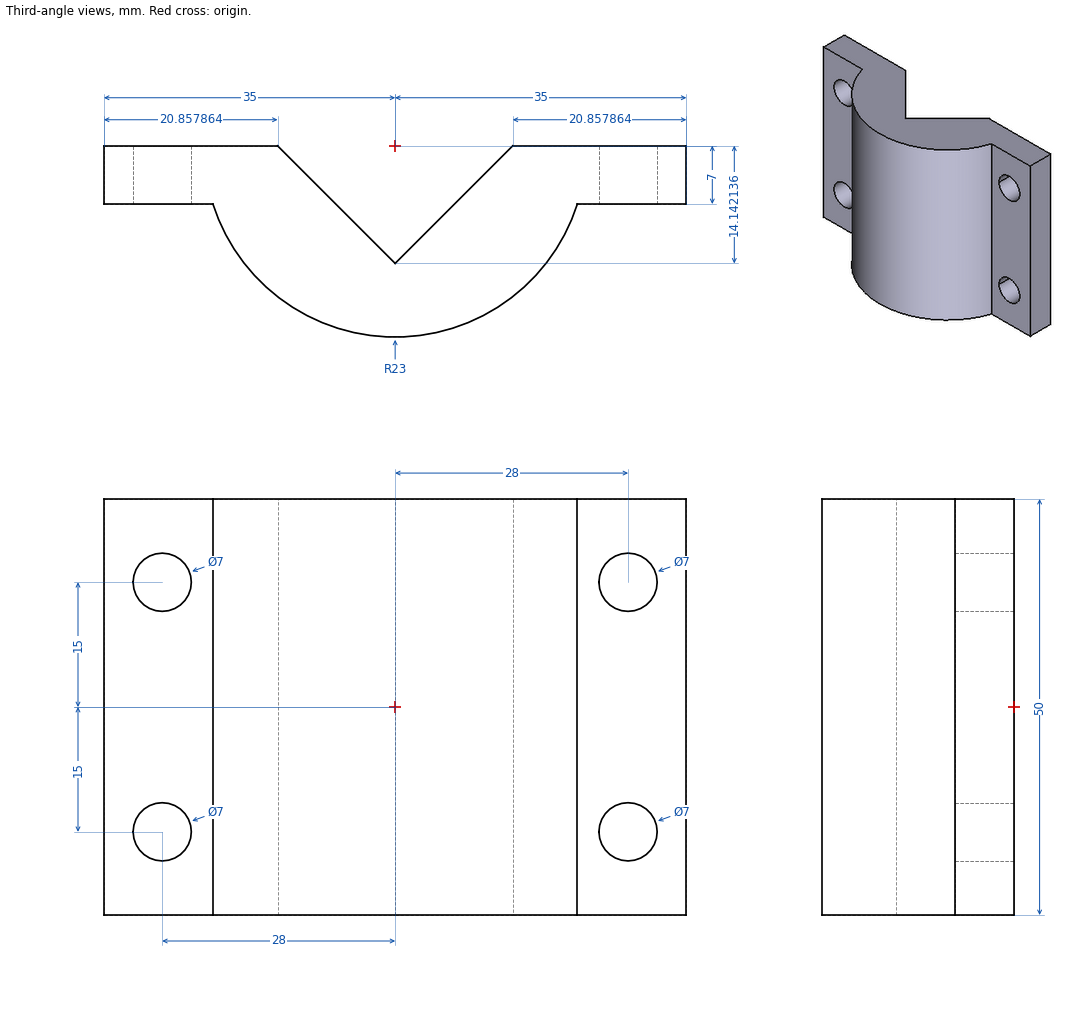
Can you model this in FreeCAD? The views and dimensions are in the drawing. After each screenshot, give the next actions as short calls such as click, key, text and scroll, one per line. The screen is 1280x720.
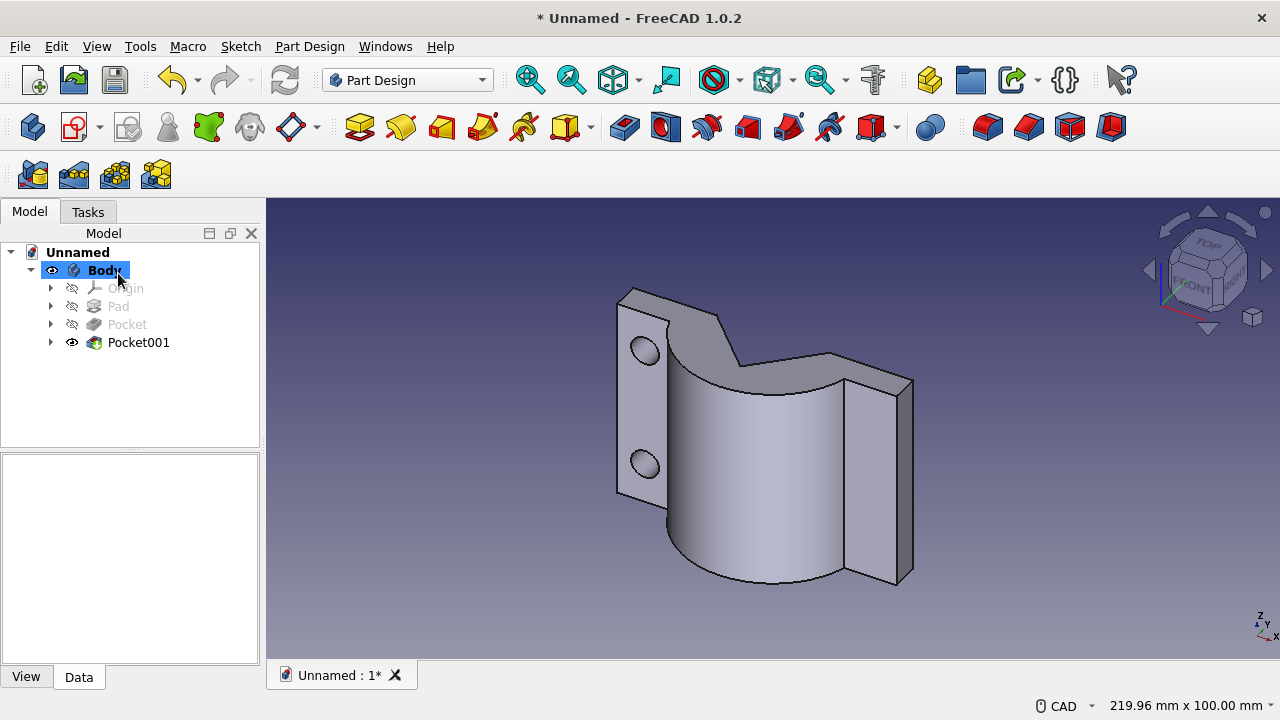
key(4)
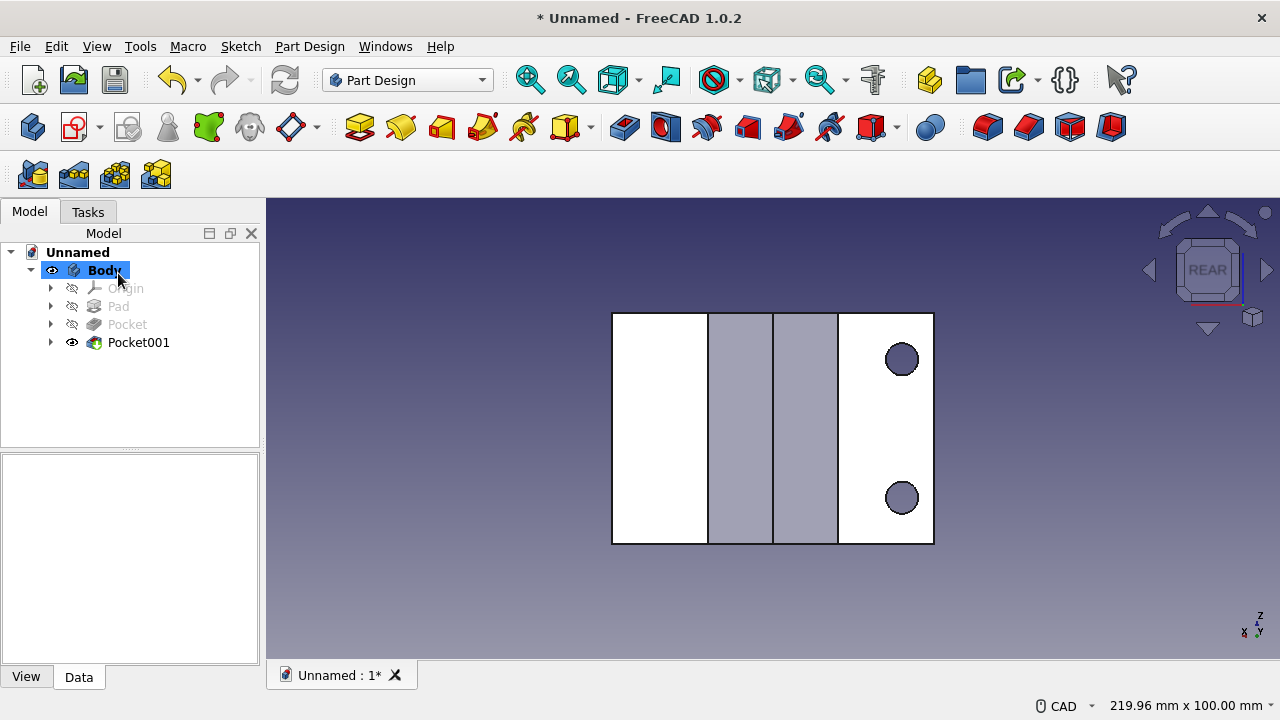
click(660, 362)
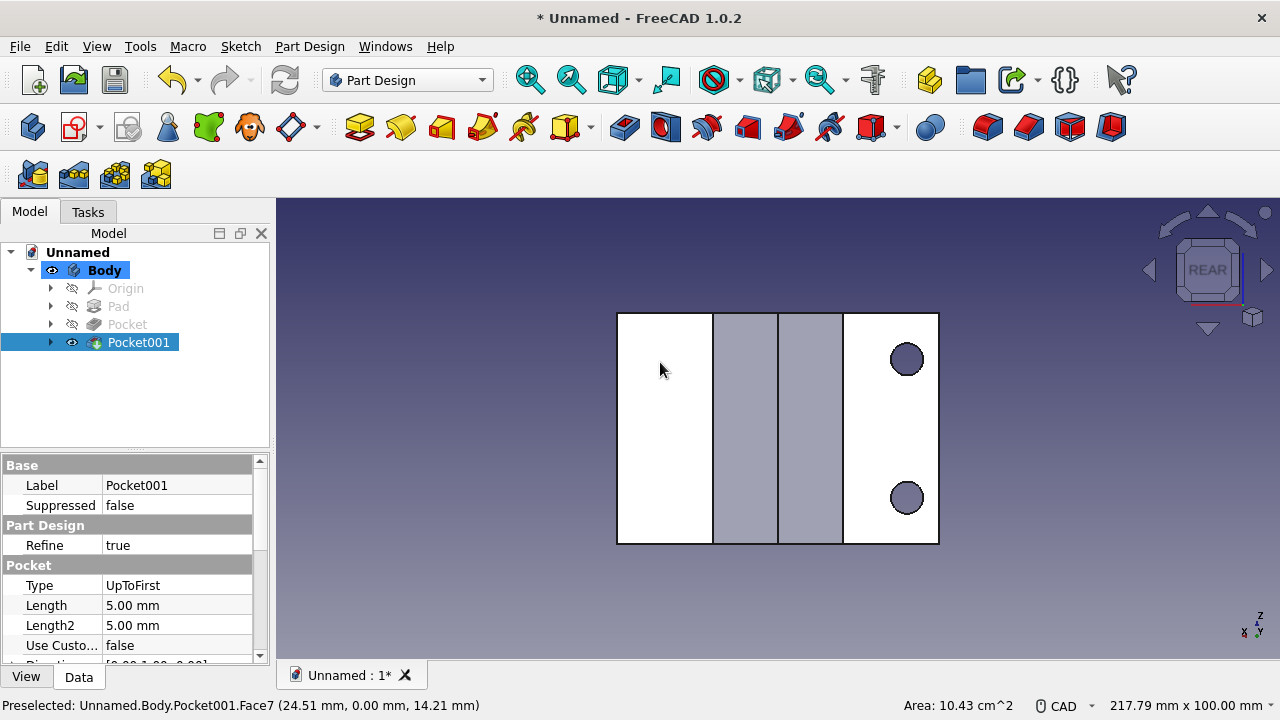
click(74, 128)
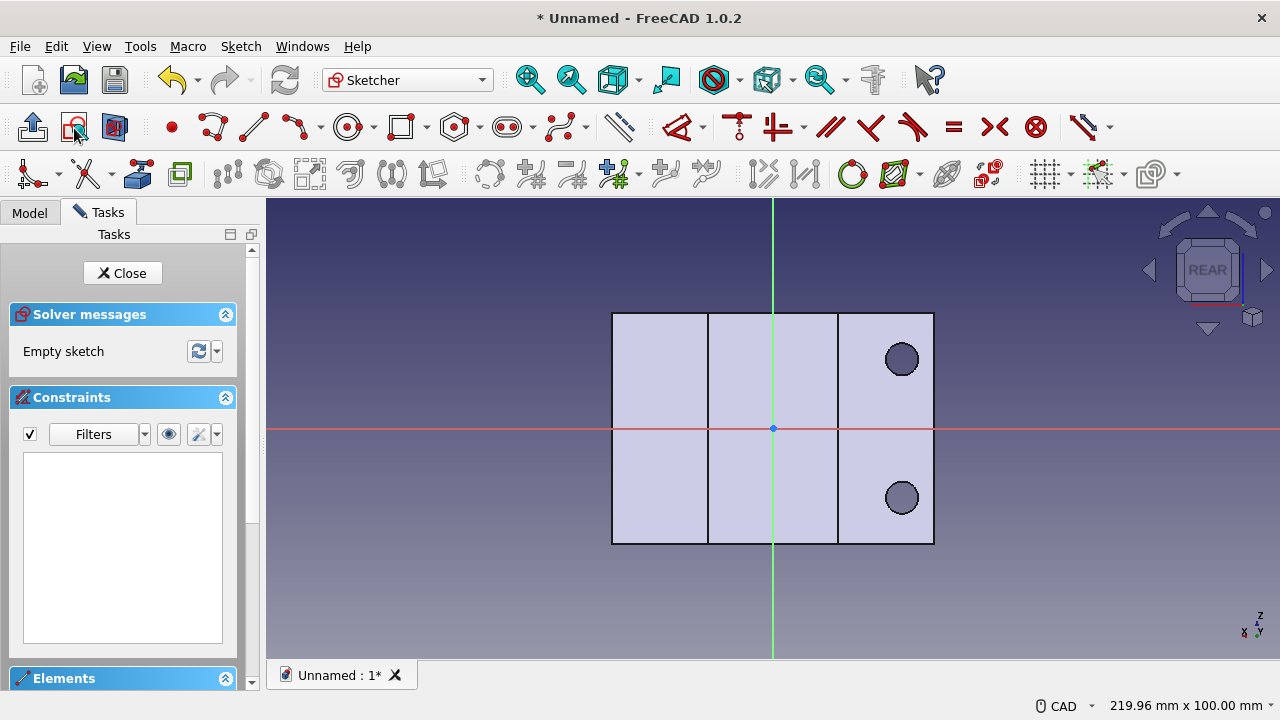
scroll(636, 351, up, 11)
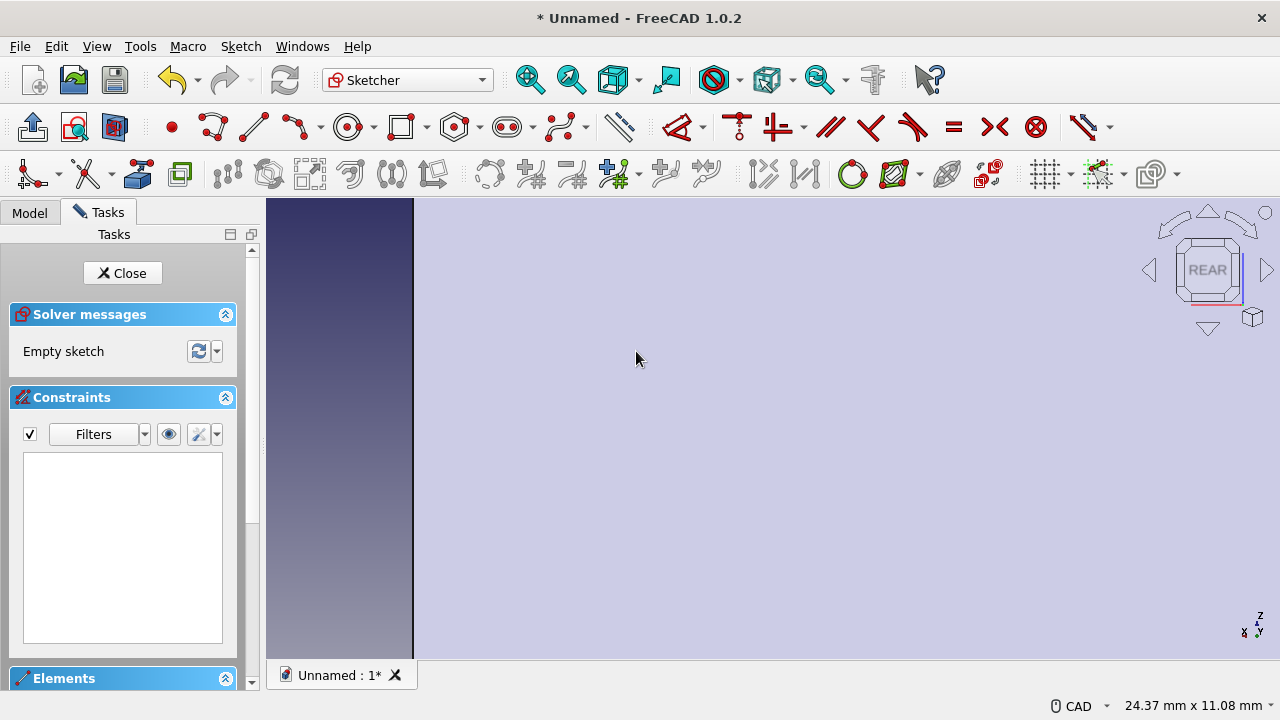
click(348, 128)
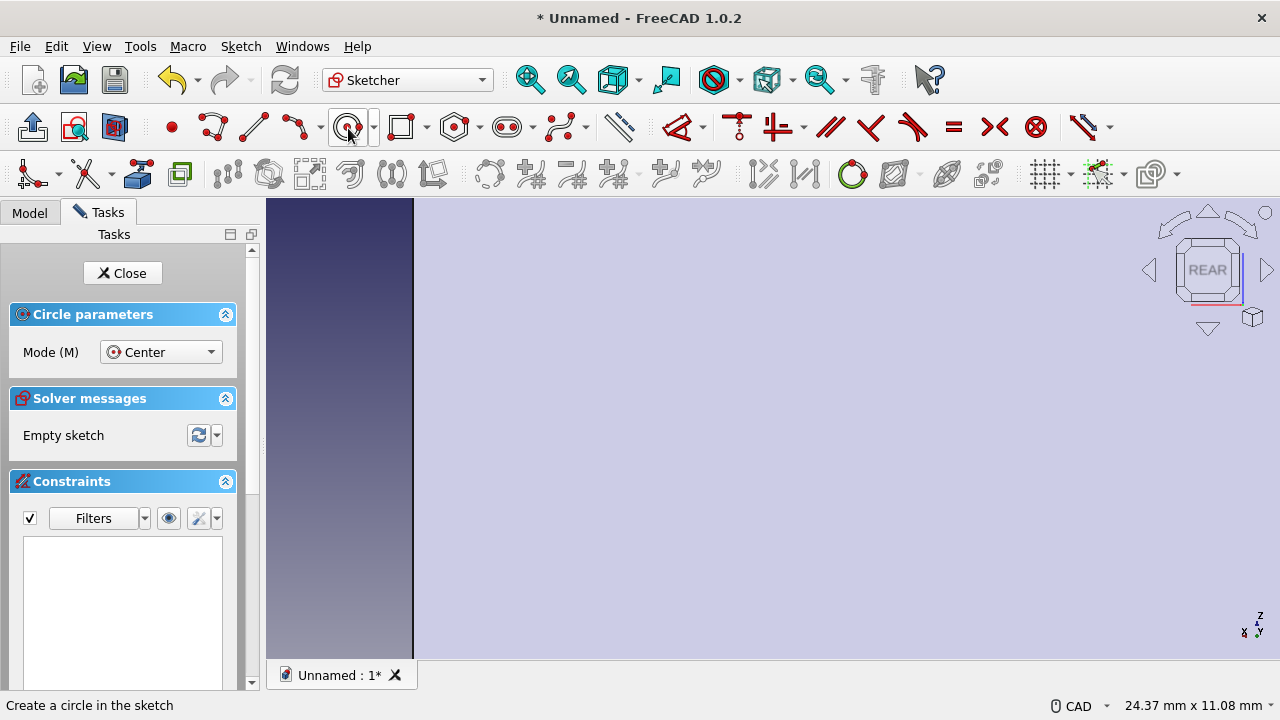
click(705, 424)
click(808, 321)
key(Escape)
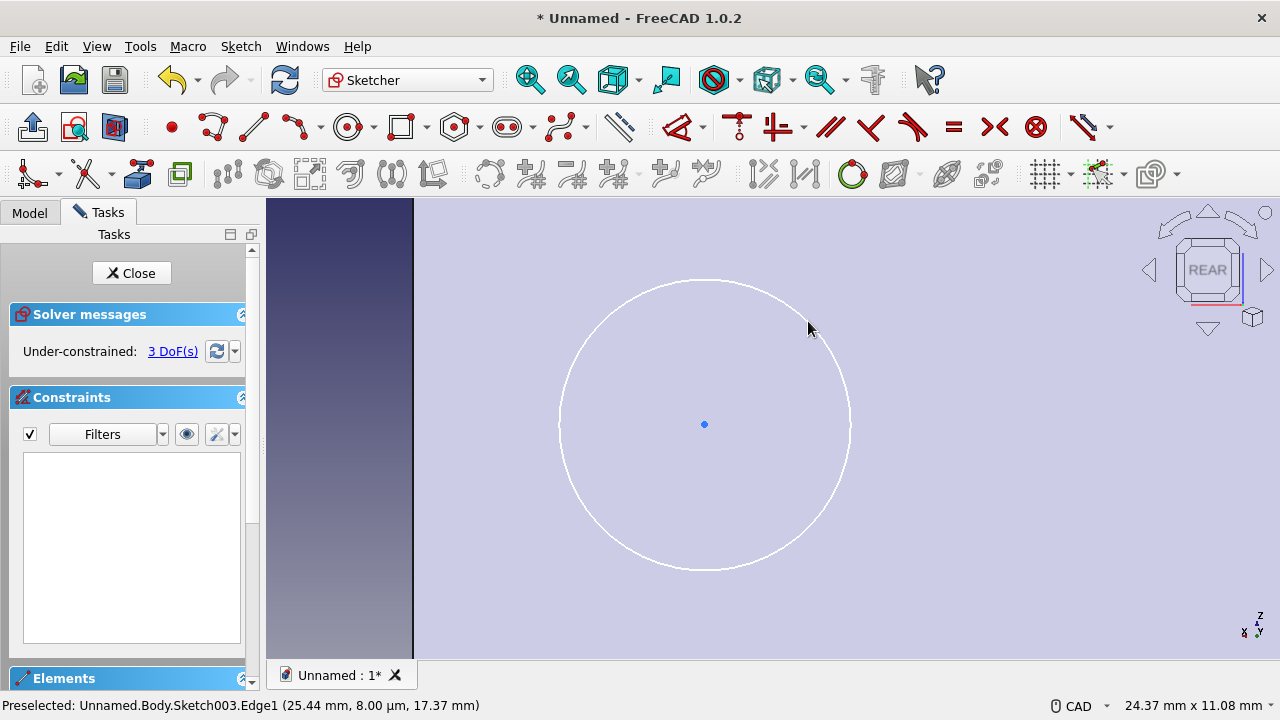
key(d)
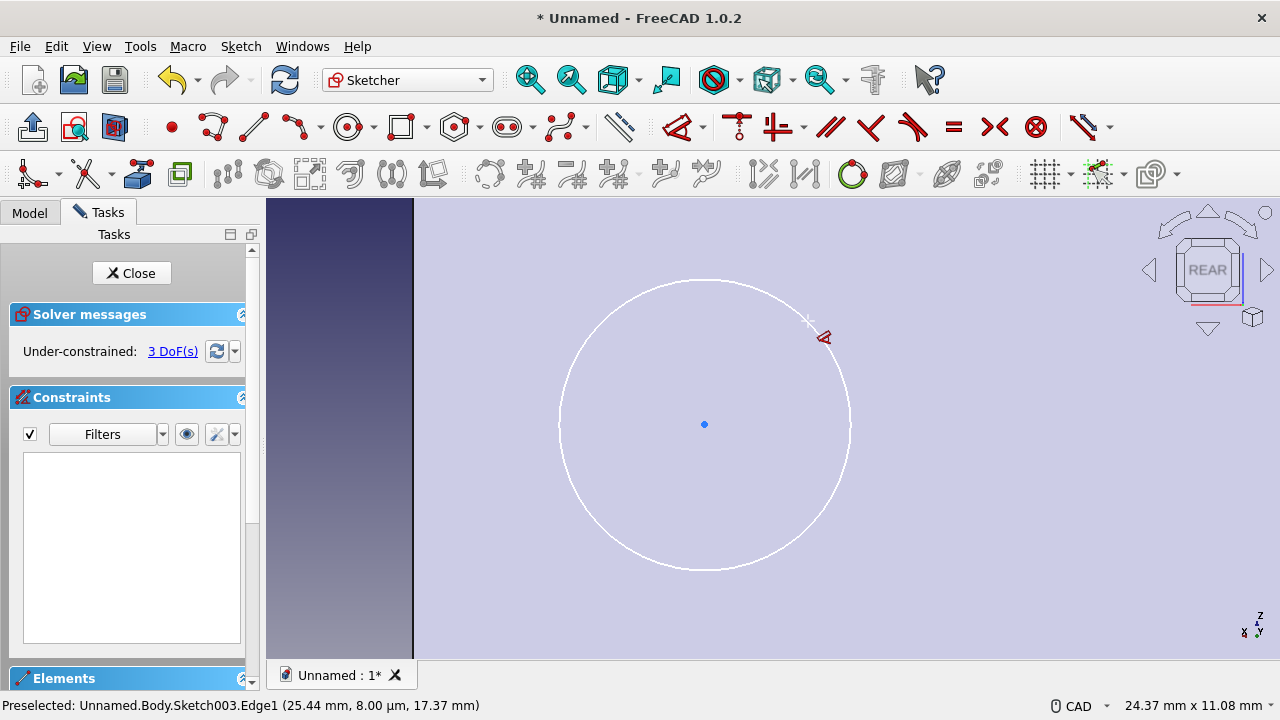
click(808, 322)
click(831, 299)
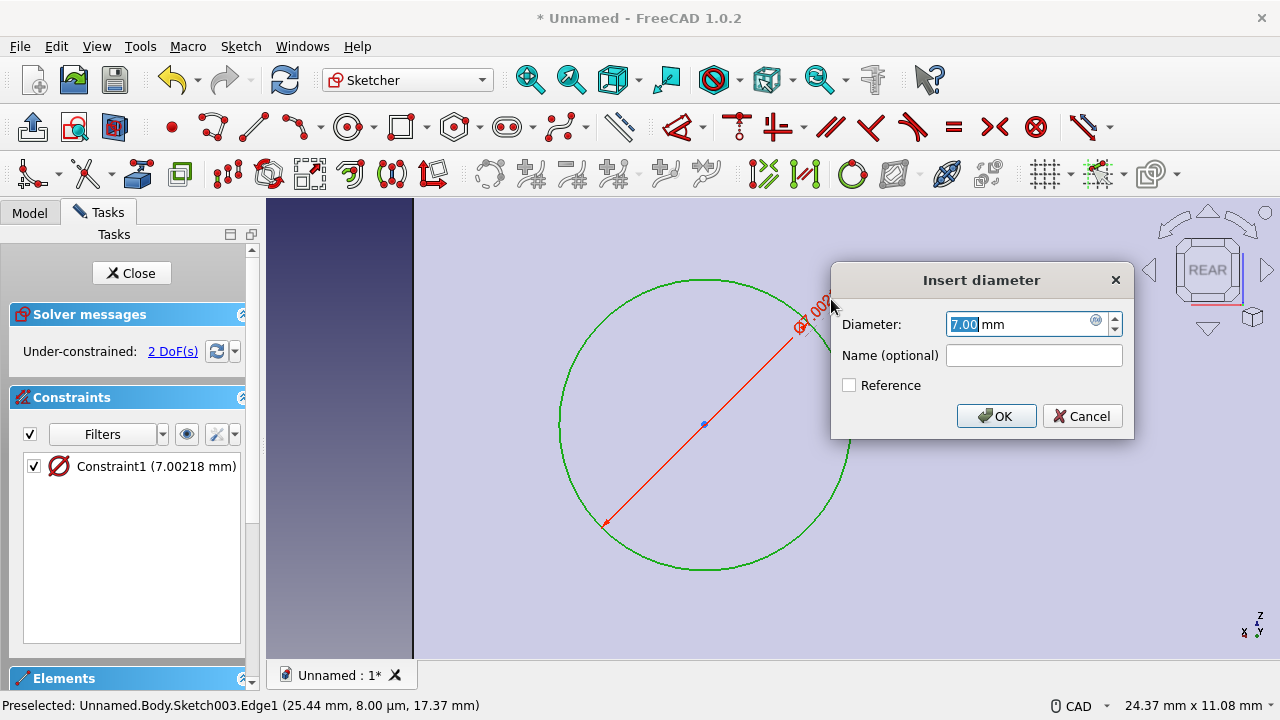
text(7)
key(Return)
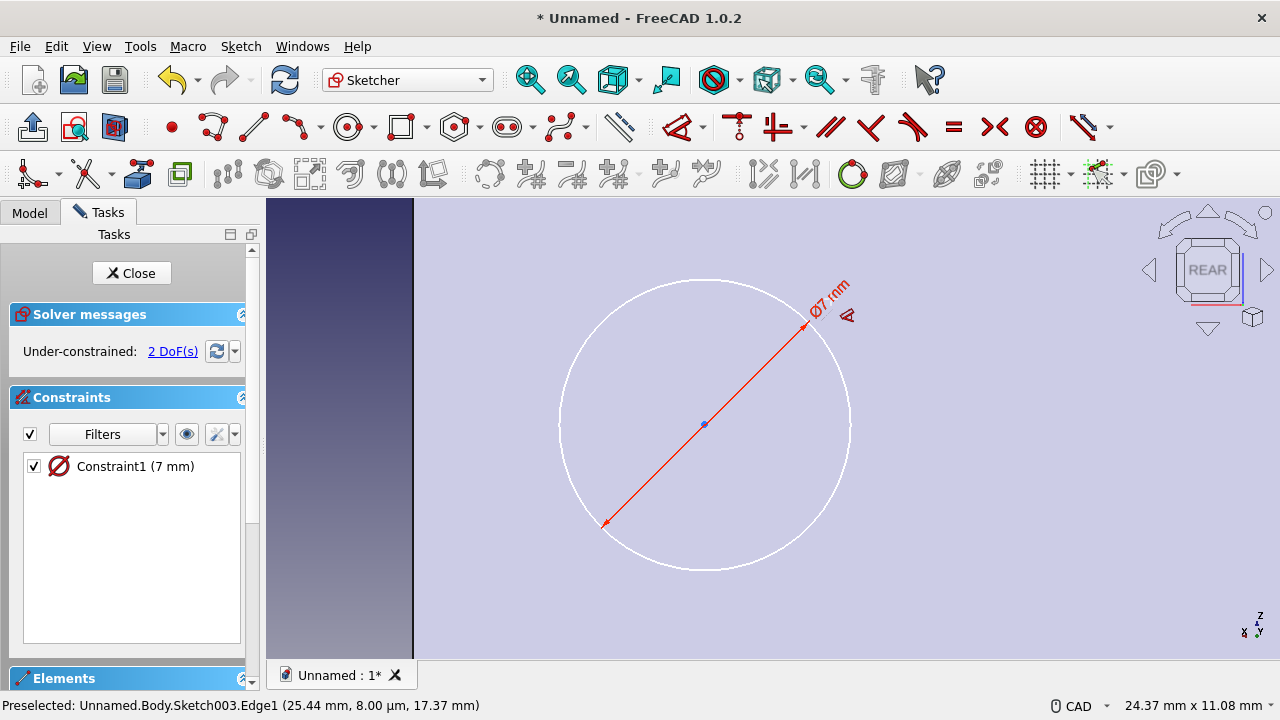
click(705, 425)
click(910, 391)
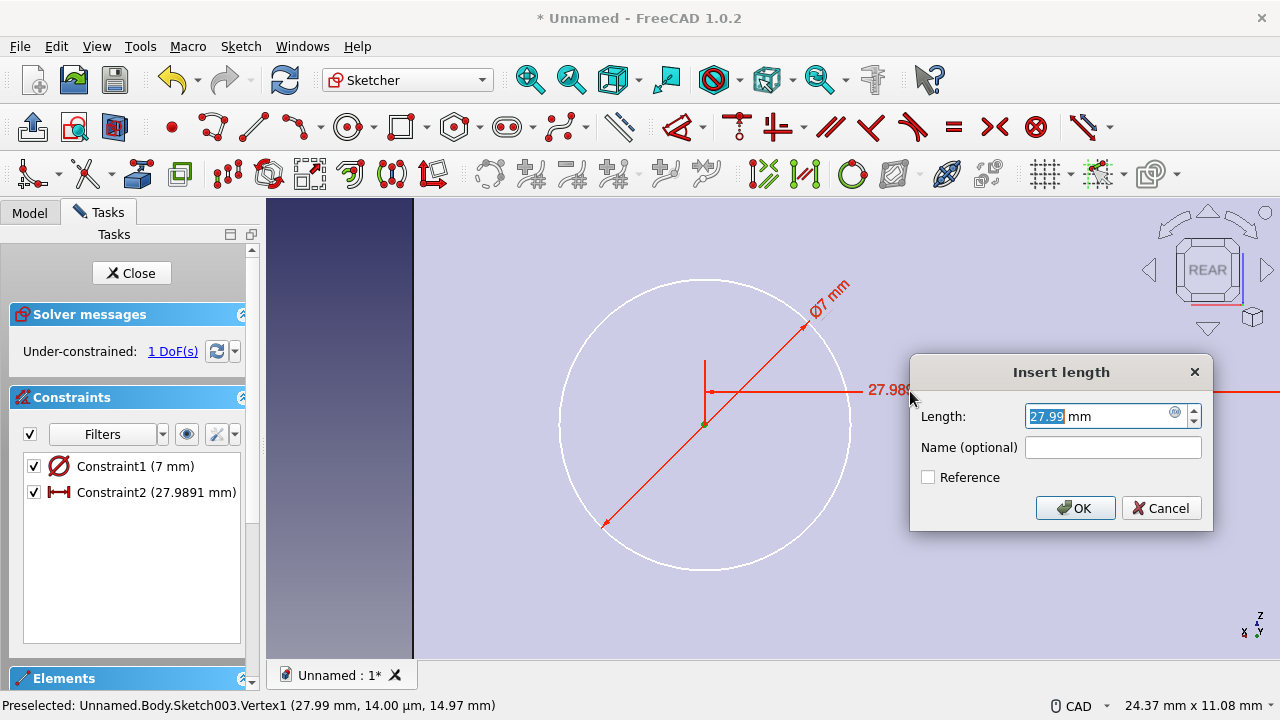
text(28)
key(Return)